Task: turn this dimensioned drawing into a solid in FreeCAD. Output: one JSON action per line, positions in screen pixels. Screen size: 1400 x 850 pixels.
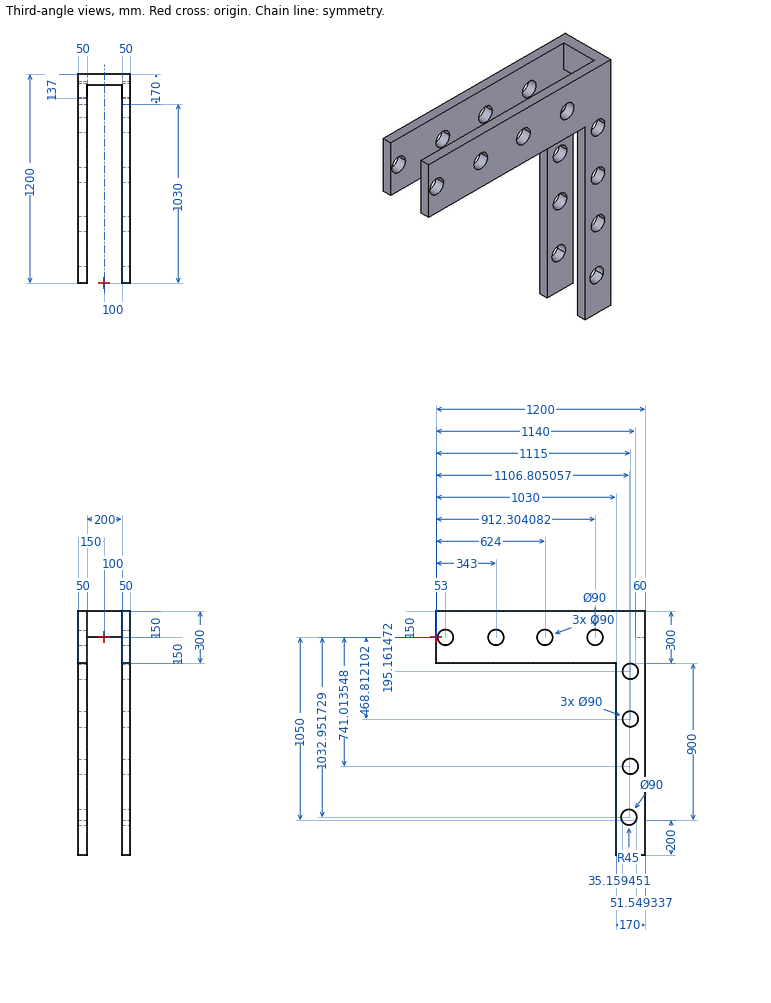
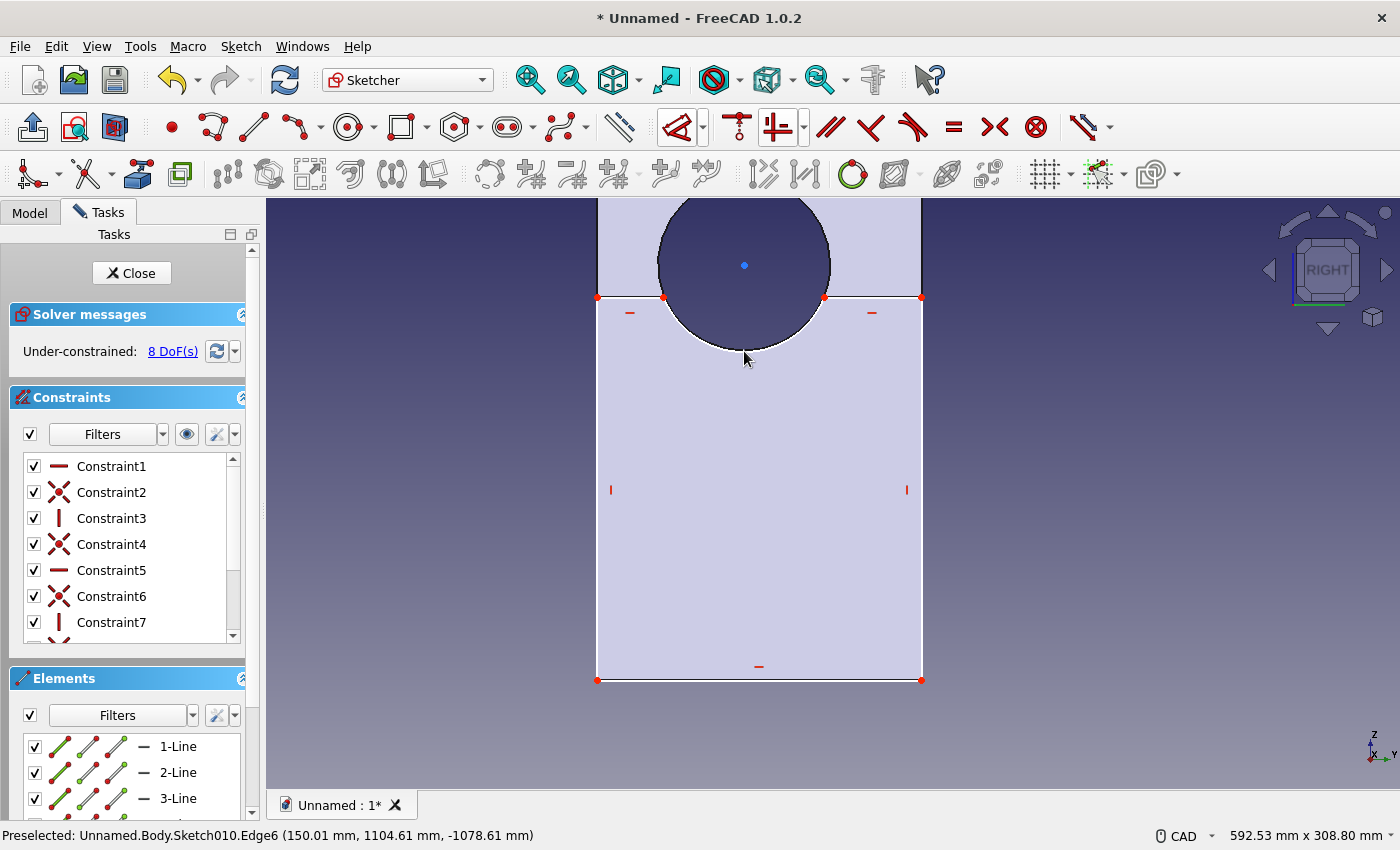
{"action": "left_click", "coordinate": [705, 342]}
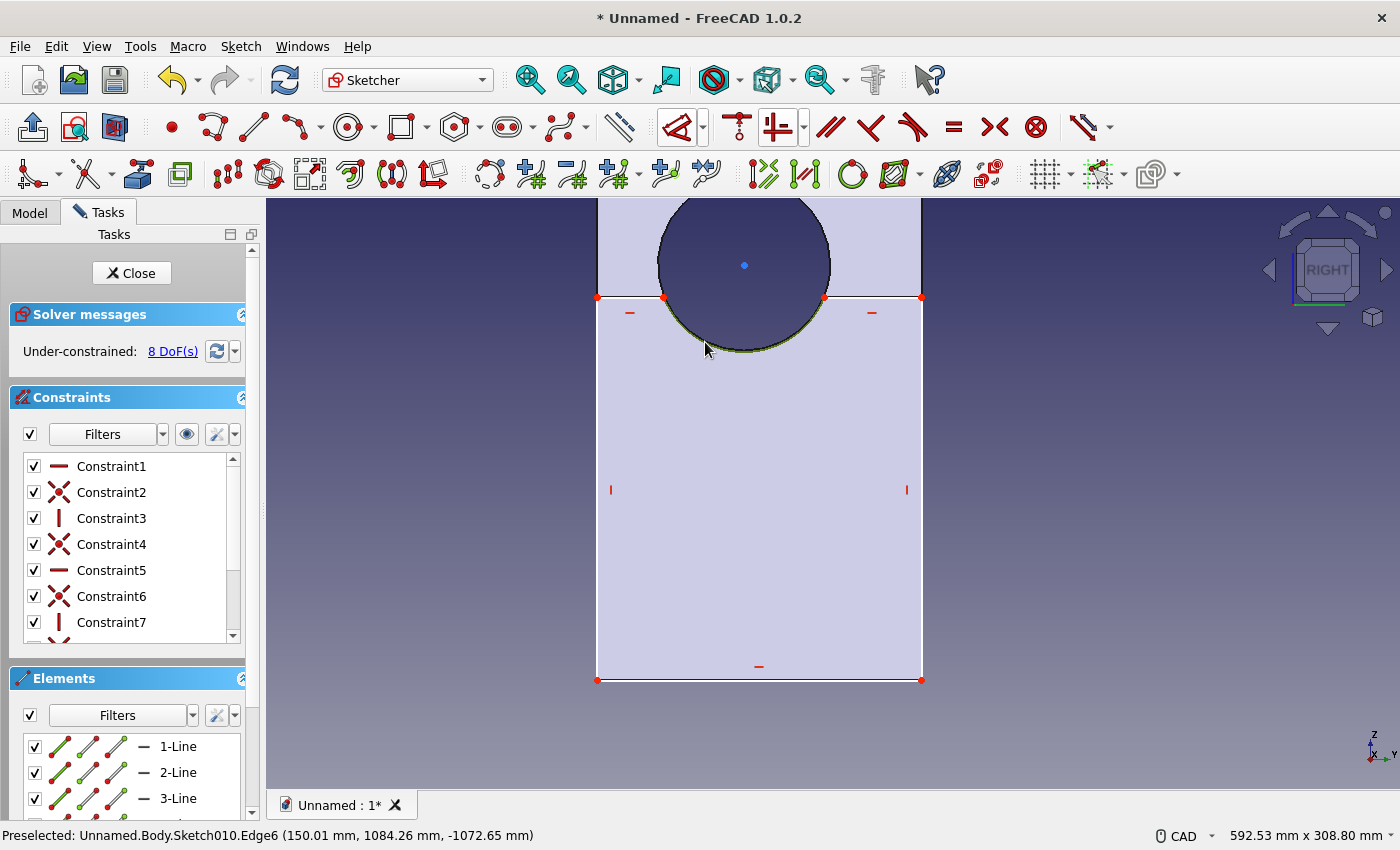
{"action": "left_click", "coordinate": [702, 128]}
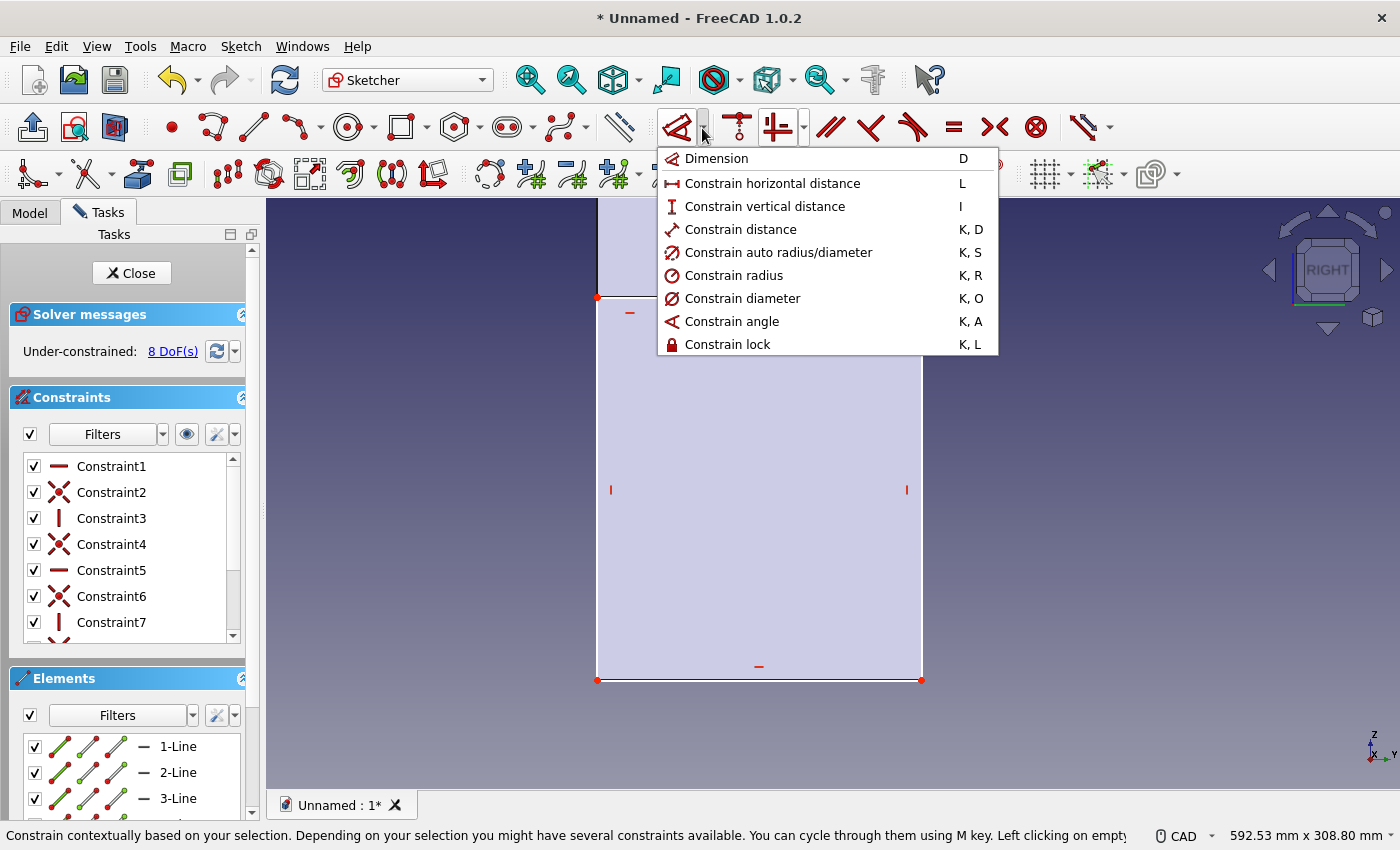
{"action": "left_click", "coordinate": [828, 276]}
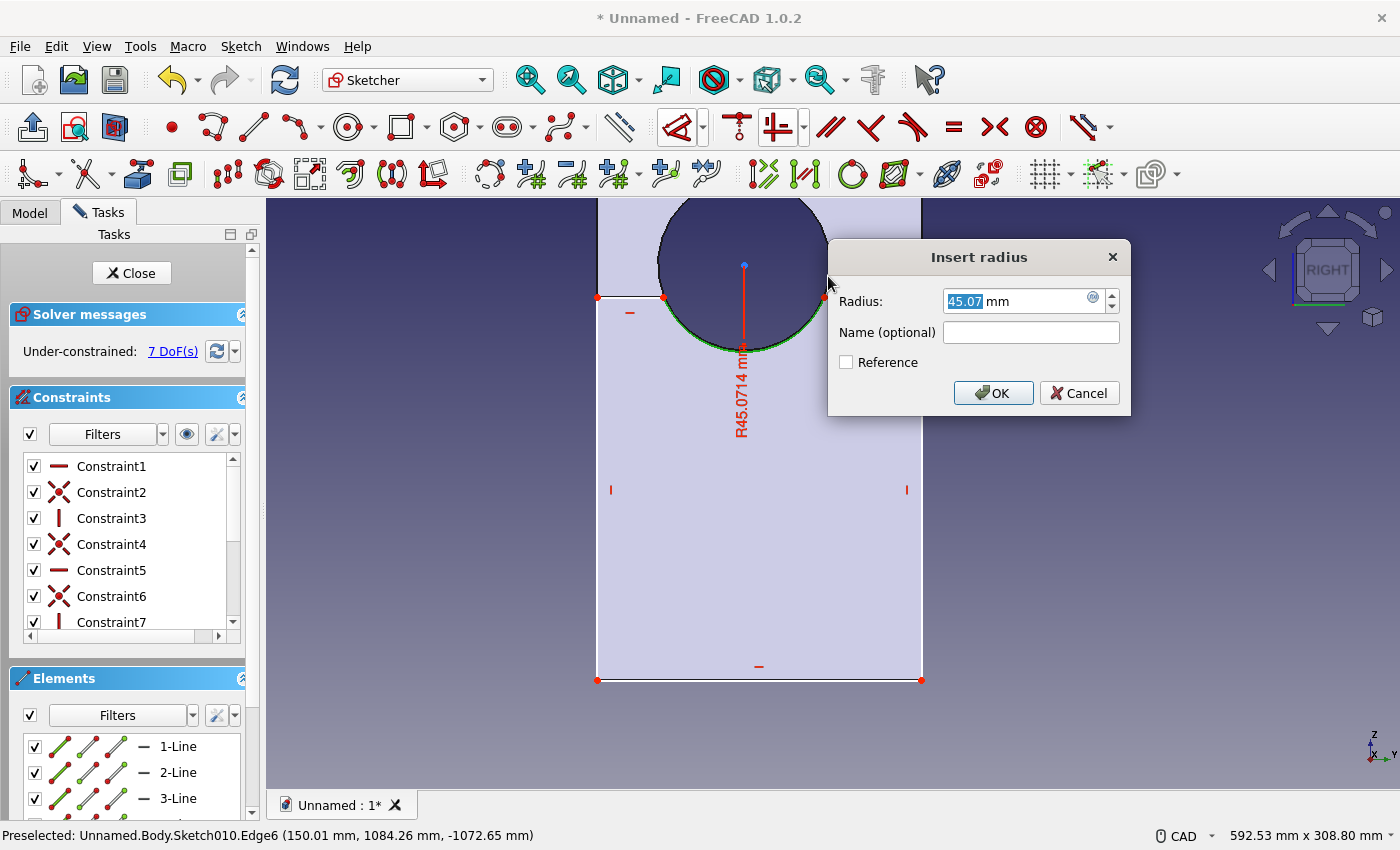
{"action": "type", "text": "45"}
{"action": "key", "text": "Return"}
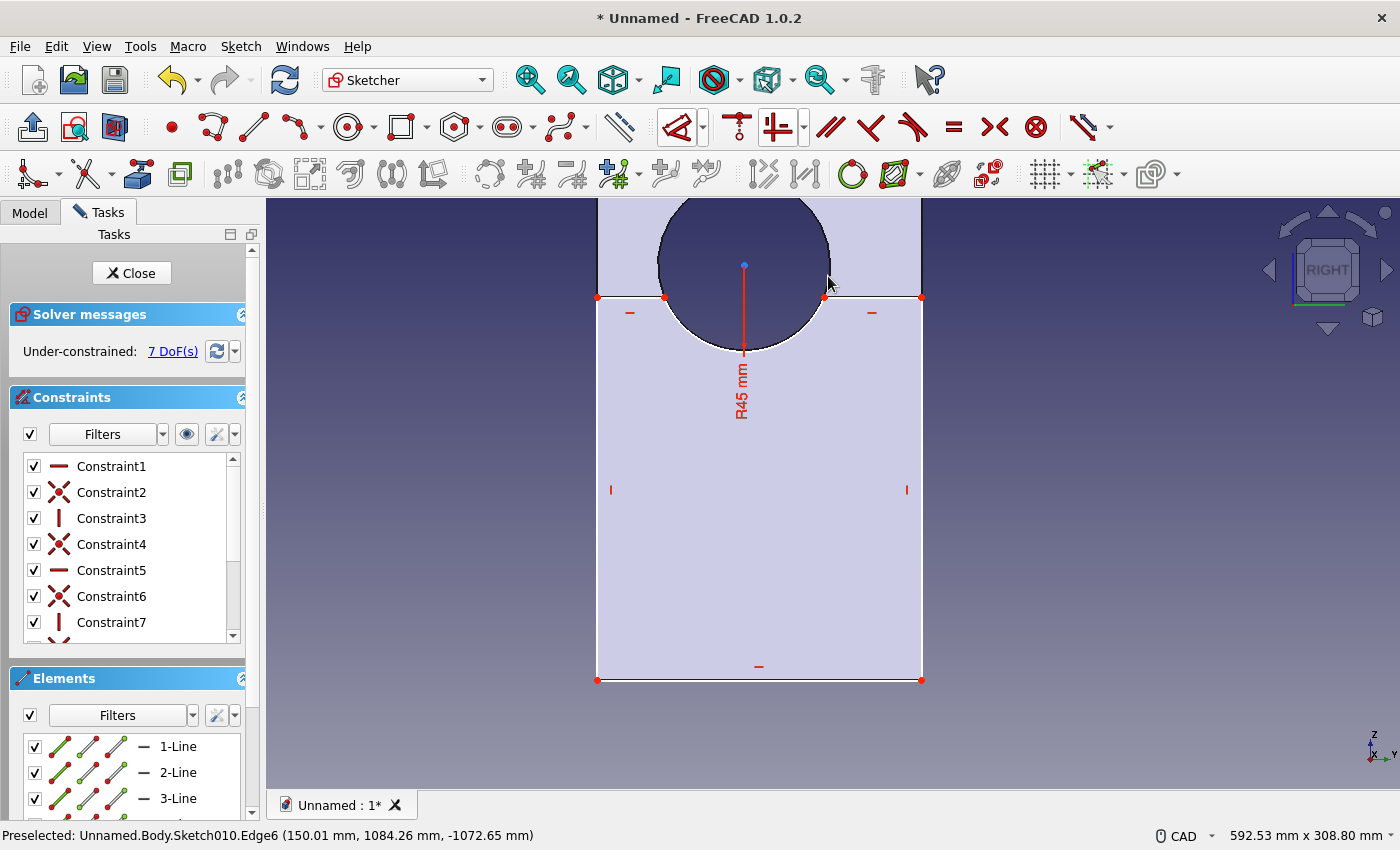
{"action": "left_click", "coordinate": [597, 413]}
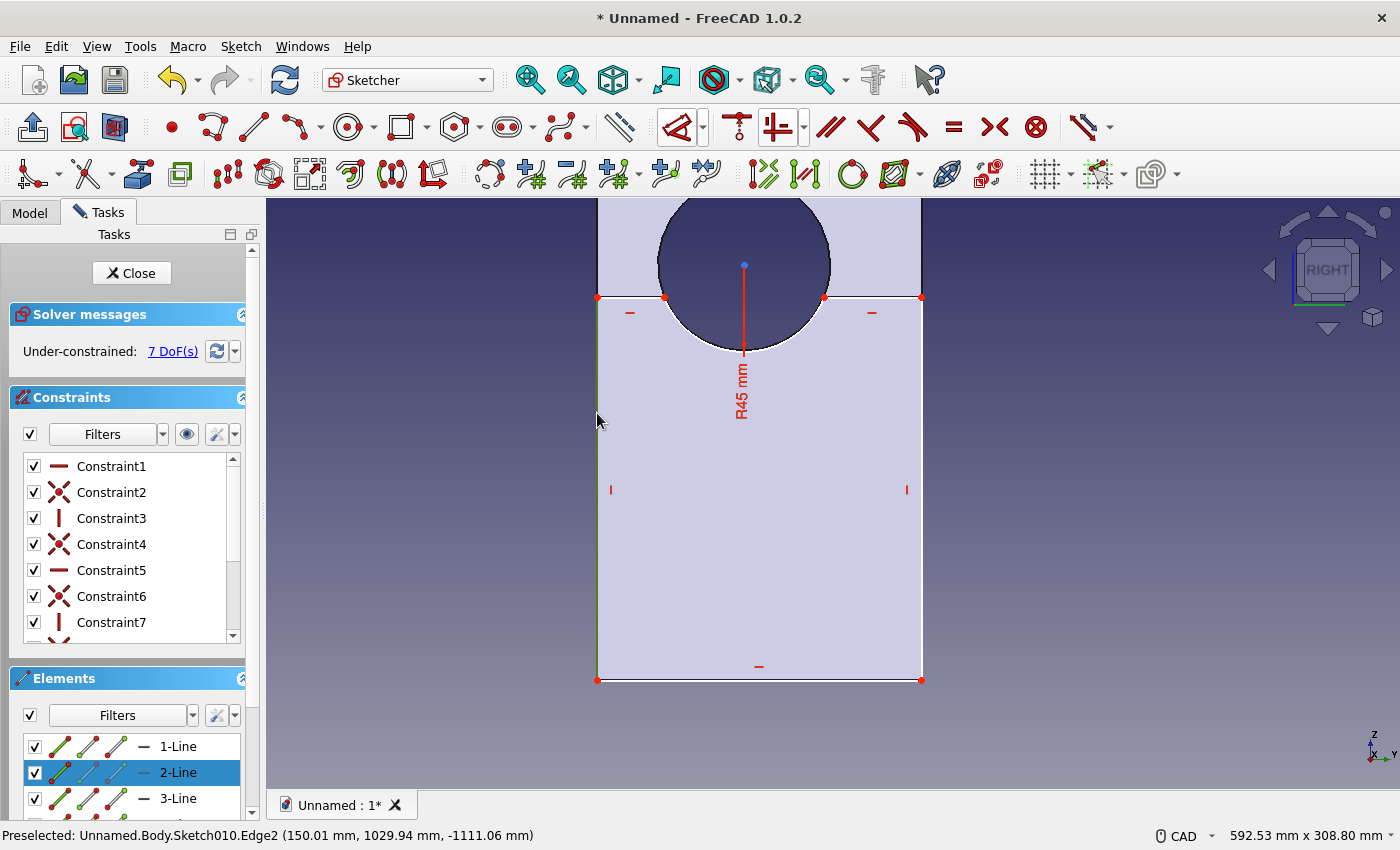
{"action": "left_click", "coordinate": [702, 128]}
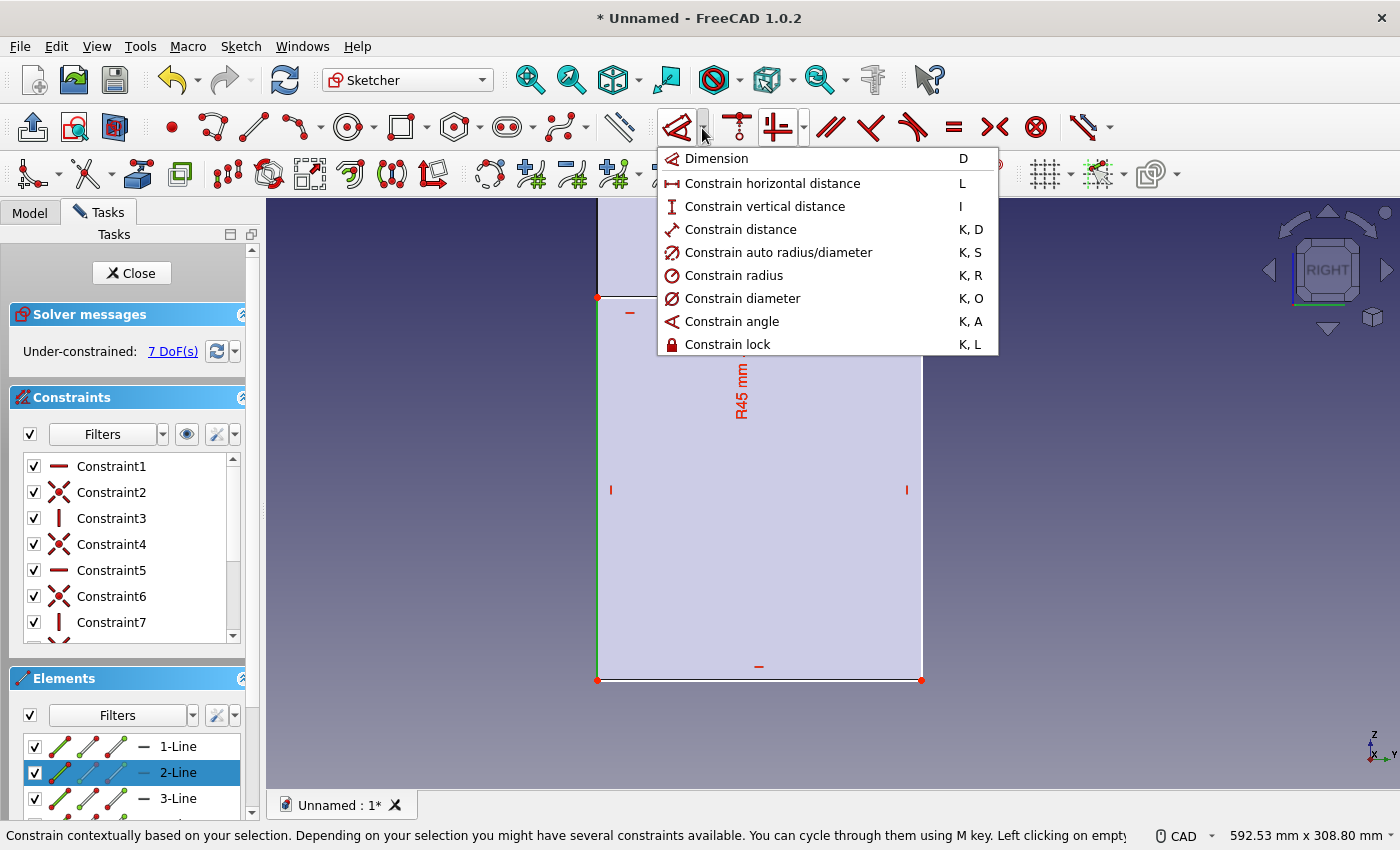
{"action": "left_click", "coordinate": [828, 206]}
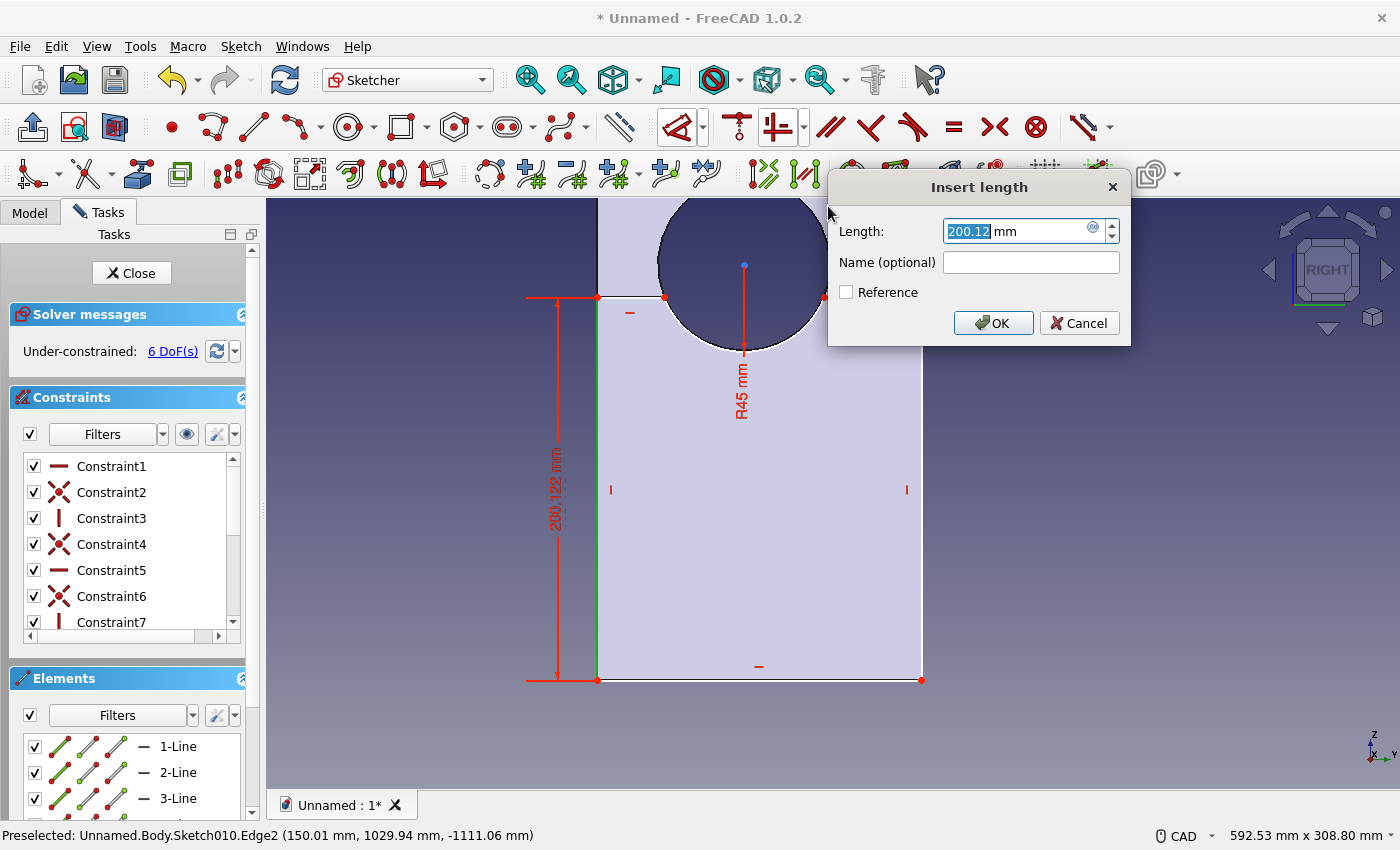
{"action": "type", "text": "200"}
{"action": "key", "text": "Return"}